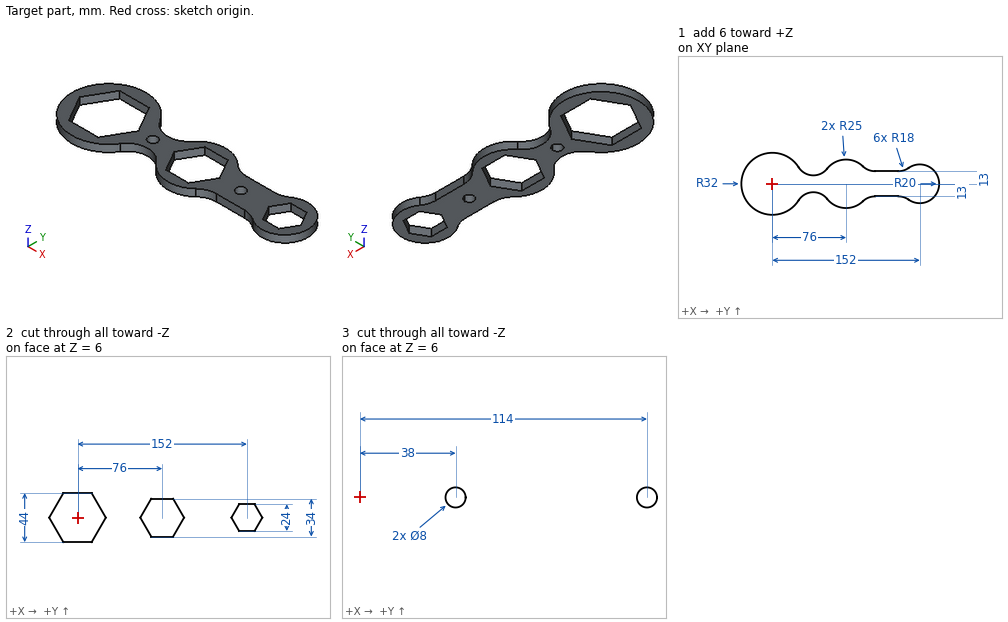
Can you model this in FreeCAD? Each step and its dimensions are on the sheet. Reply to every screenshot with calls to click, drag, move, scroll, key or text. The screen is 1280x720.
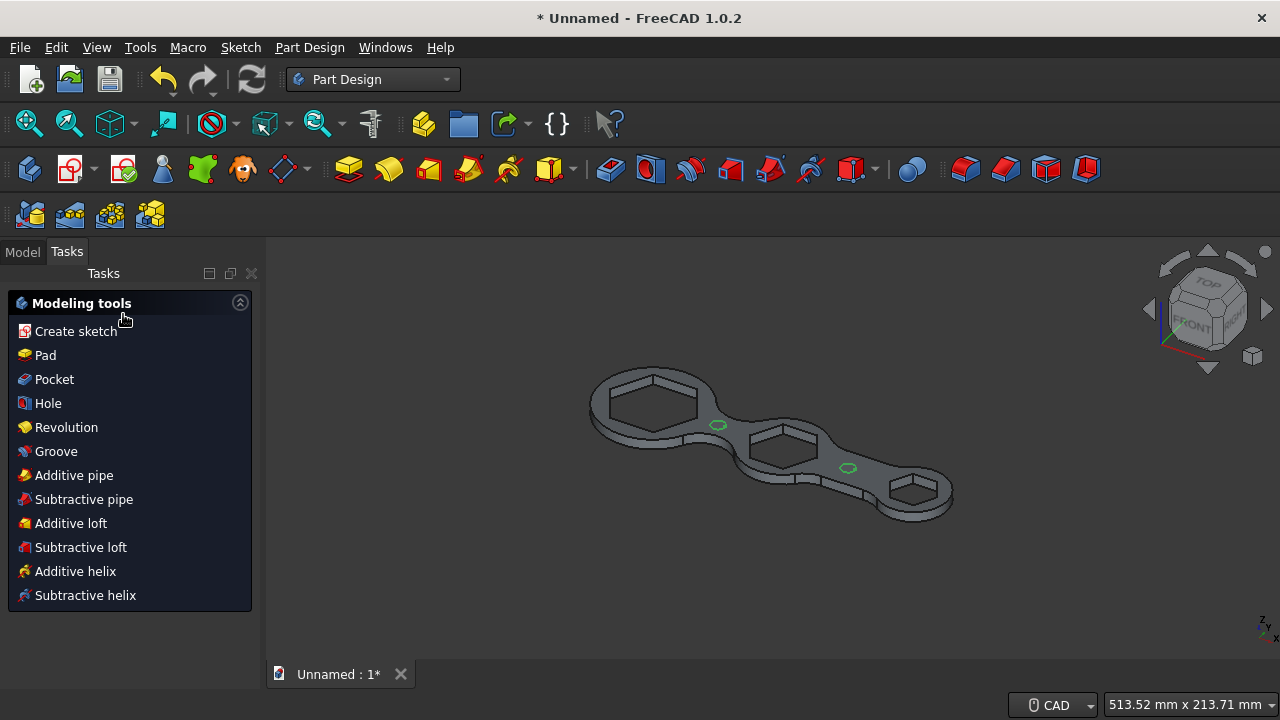
click(612, 170)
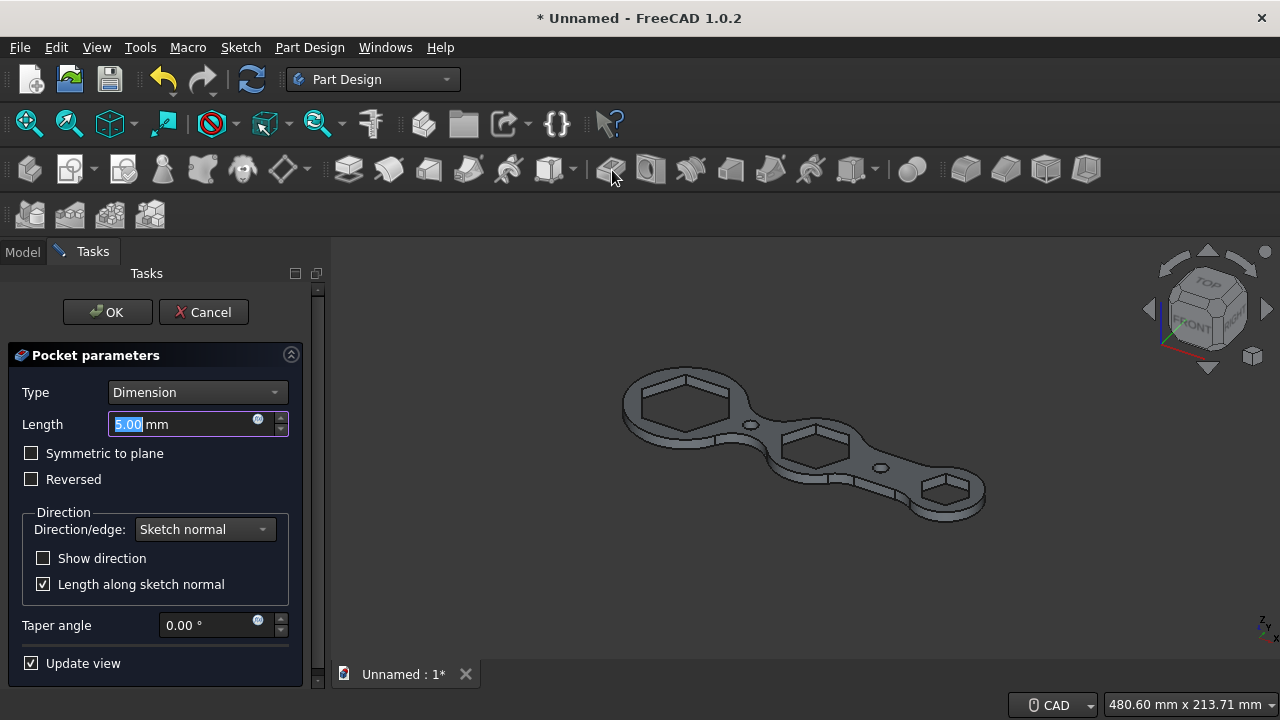
click(198, 392)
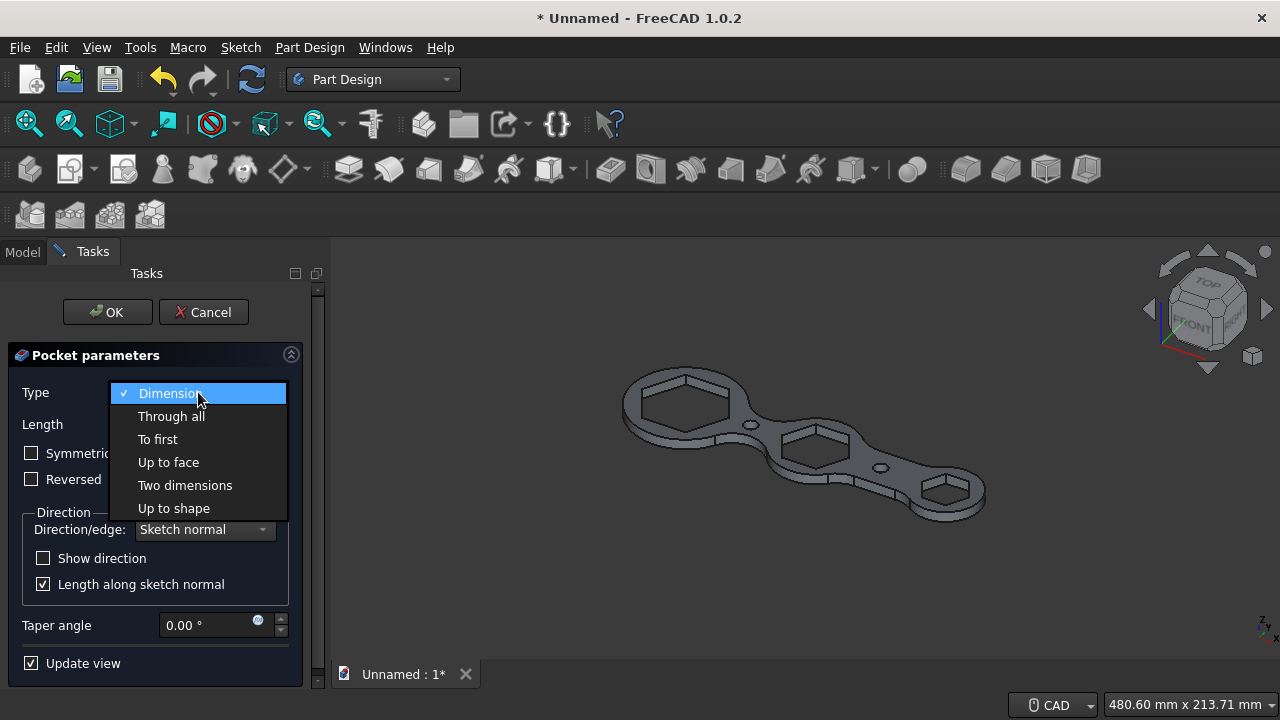
click(198, 416)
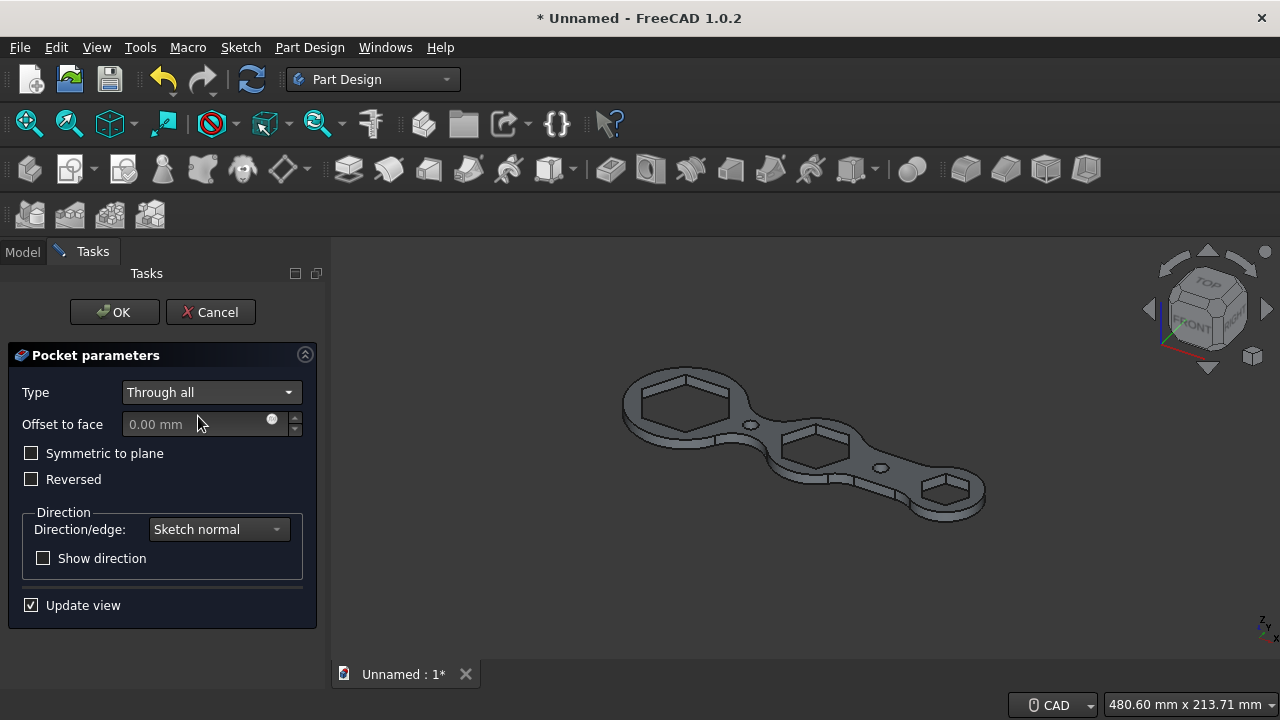
click(115, 312)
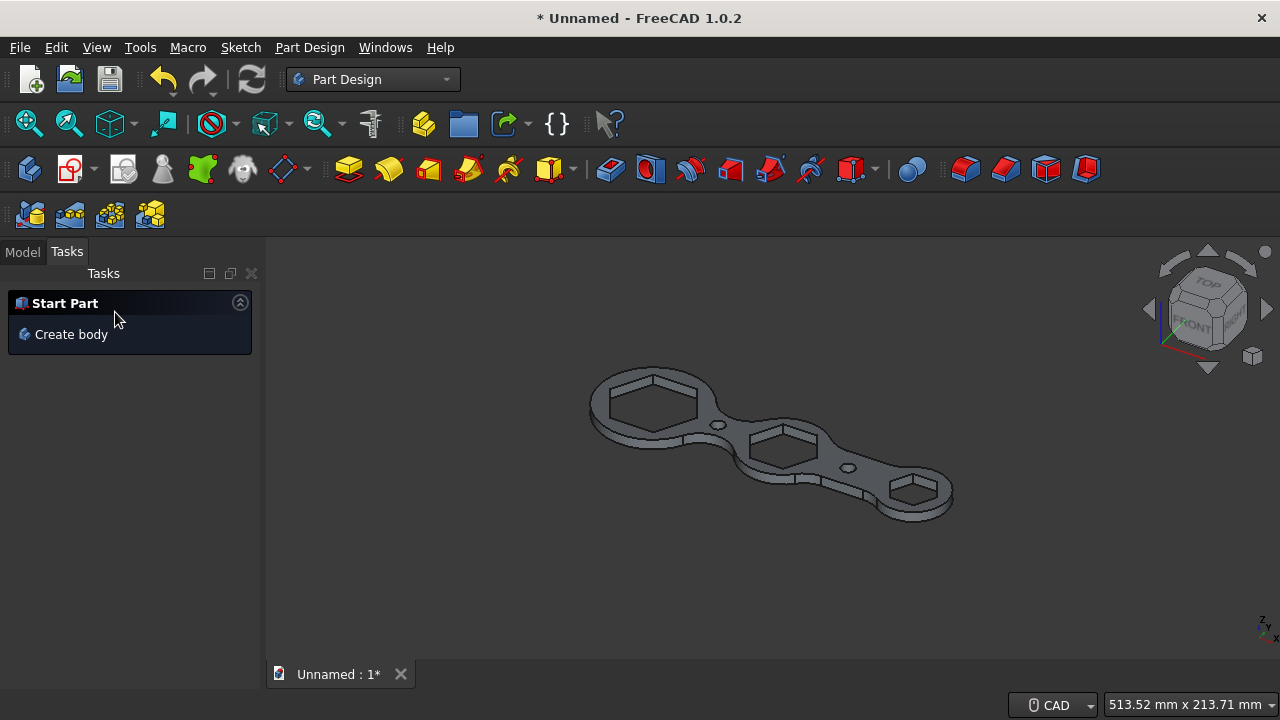
key(0)